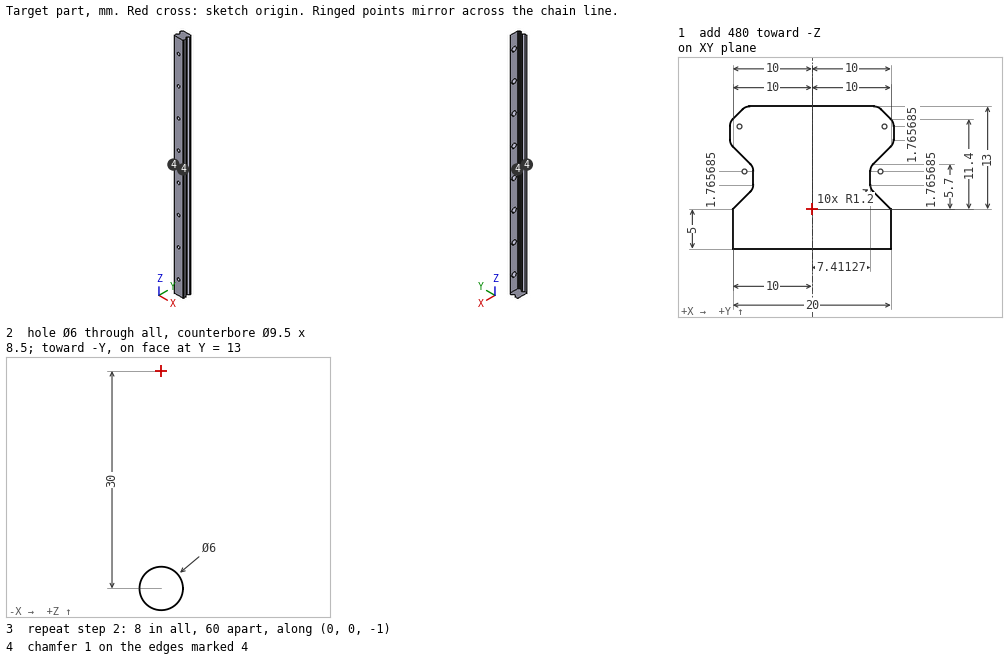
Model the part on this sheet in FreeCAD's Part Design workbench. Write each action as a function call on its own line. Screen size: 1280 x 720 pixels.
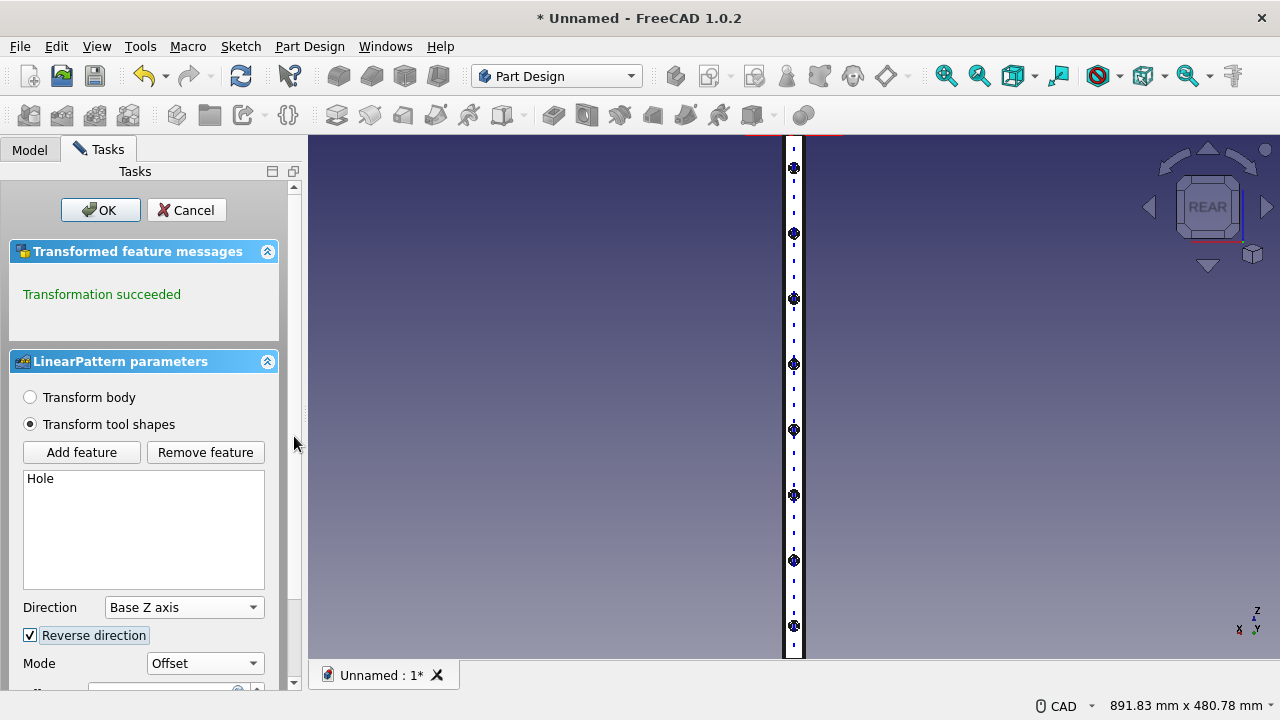
click(101, 210)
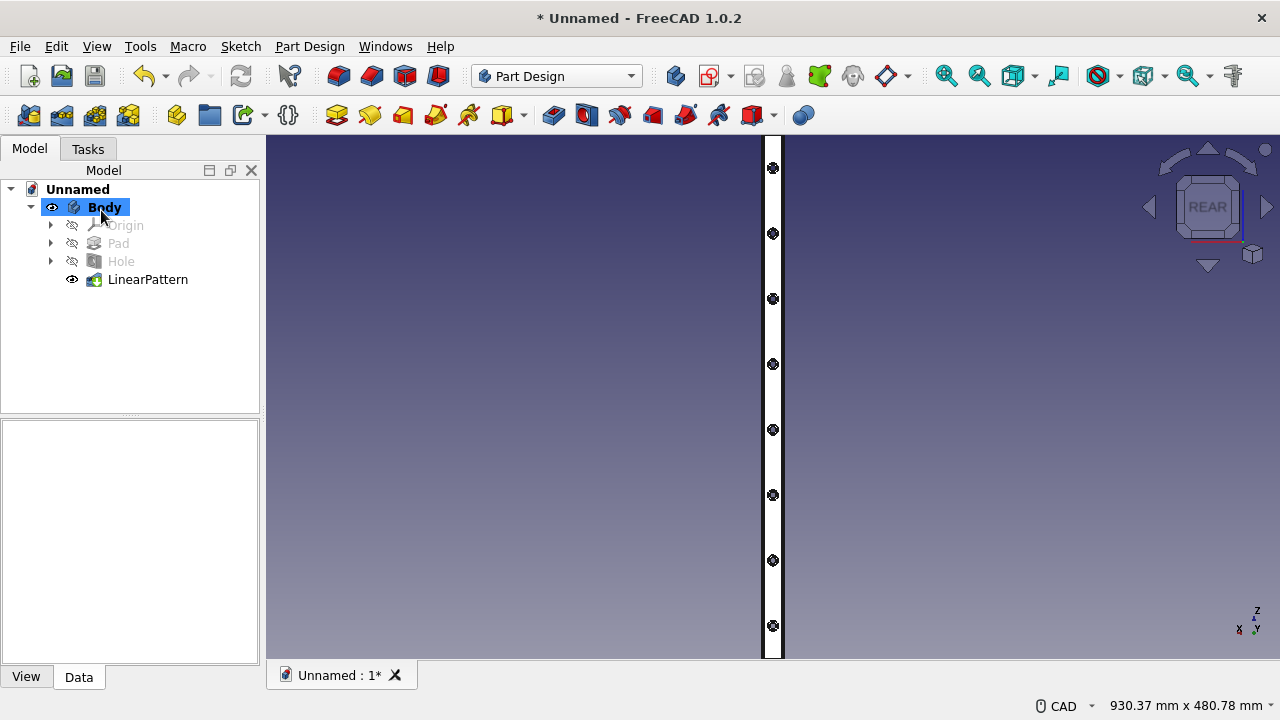
click(947, 76)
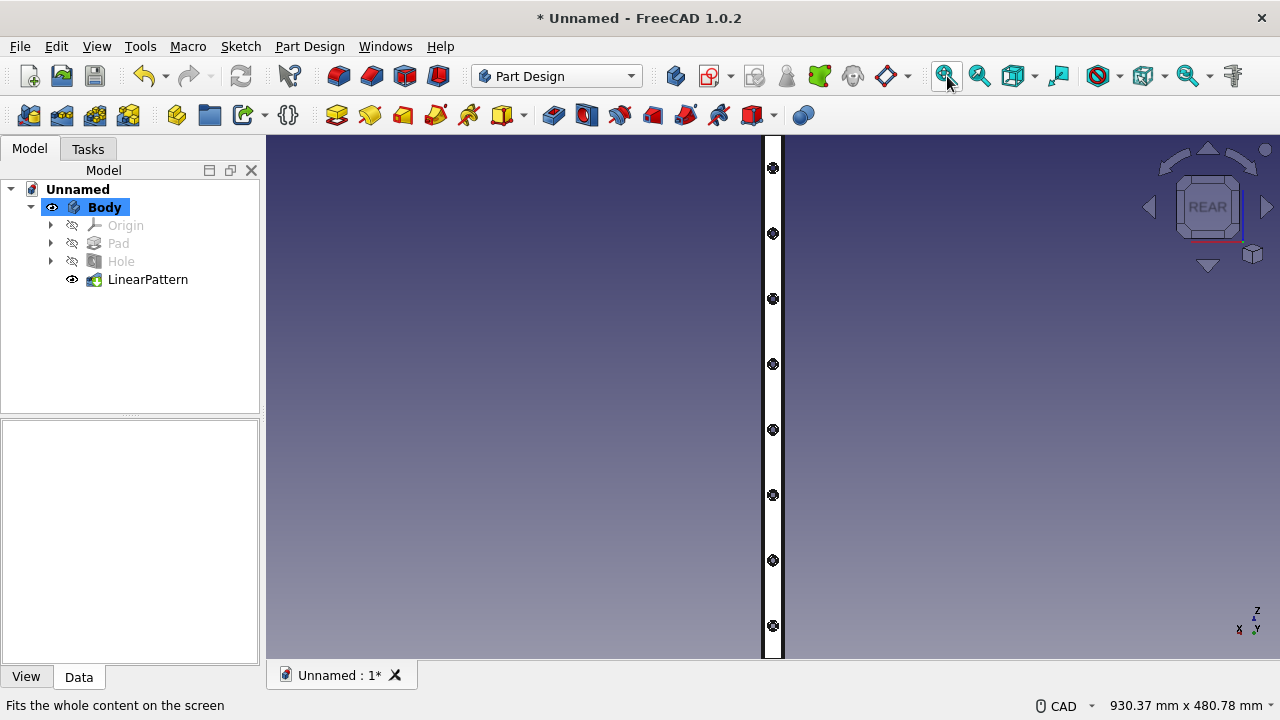
key(0)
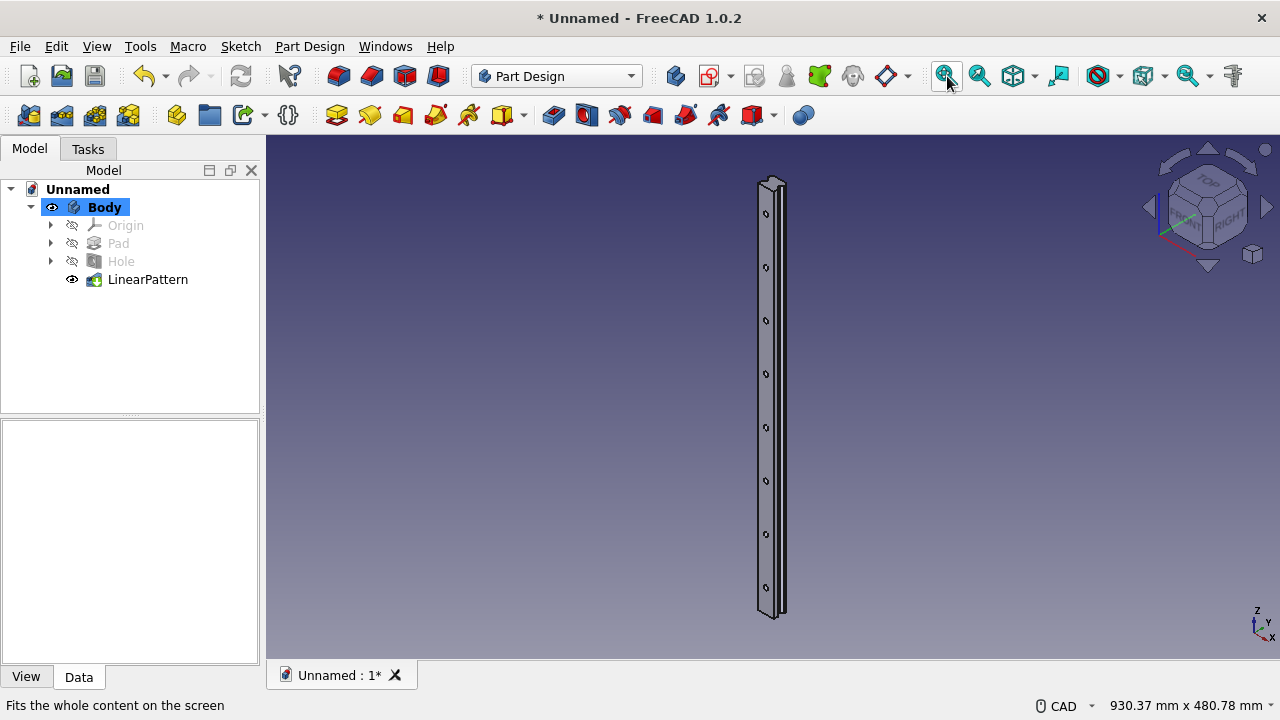
click(774, 404)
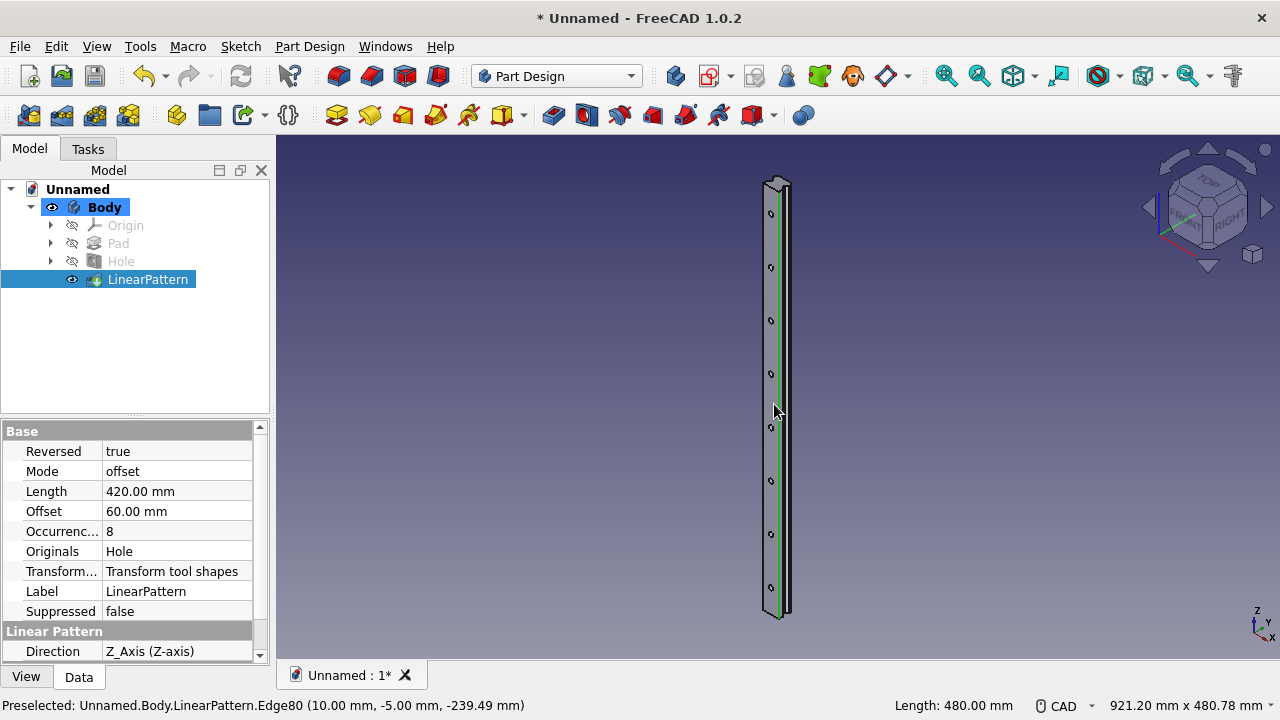
key(2)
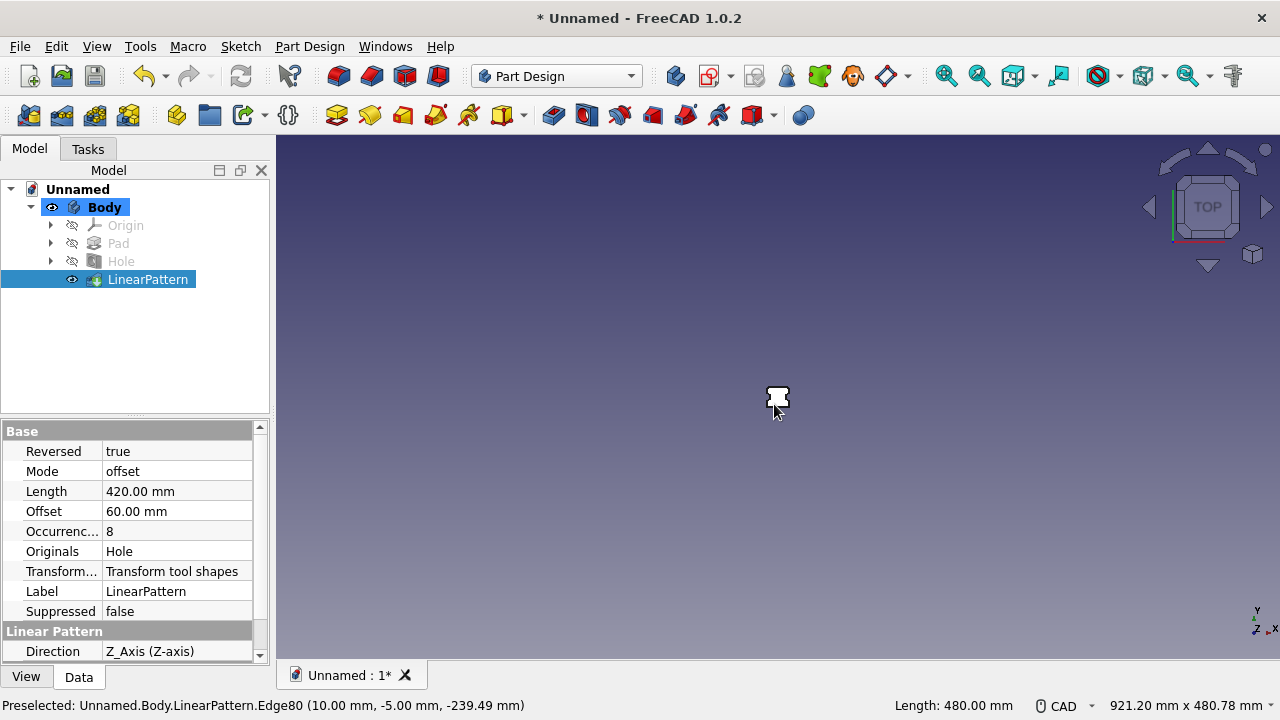
key(v)
key(f)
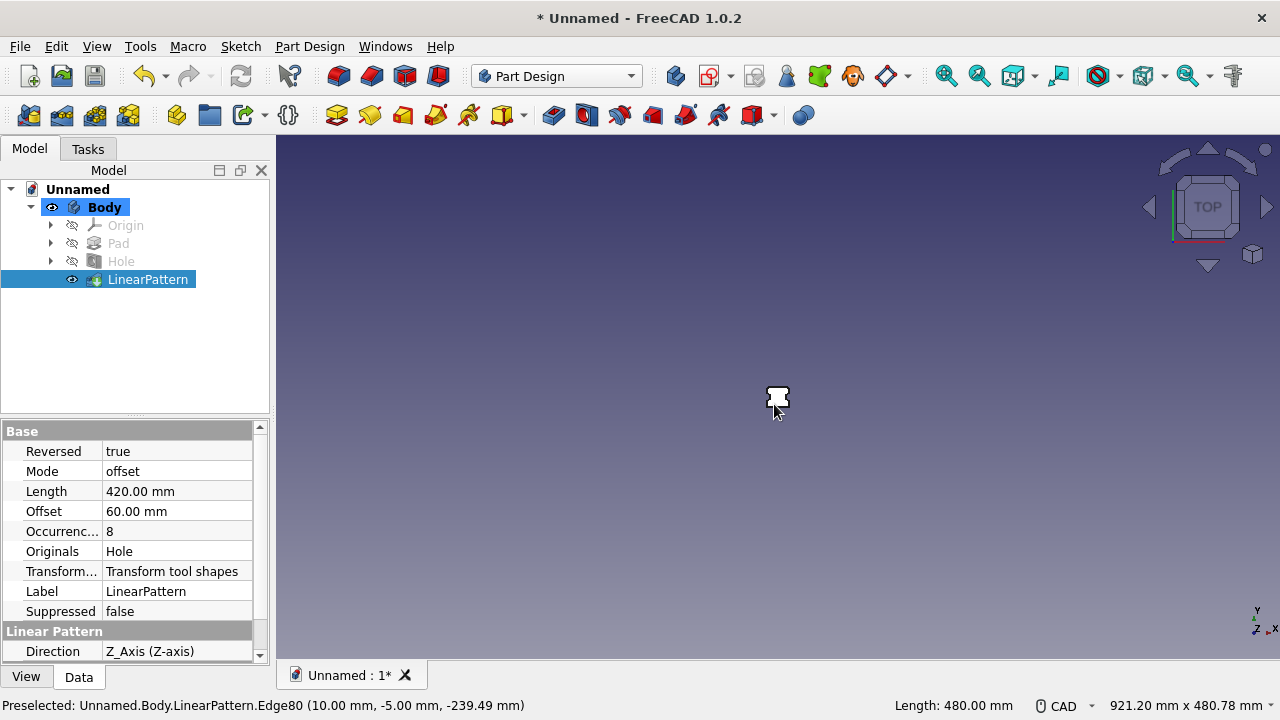
key(1)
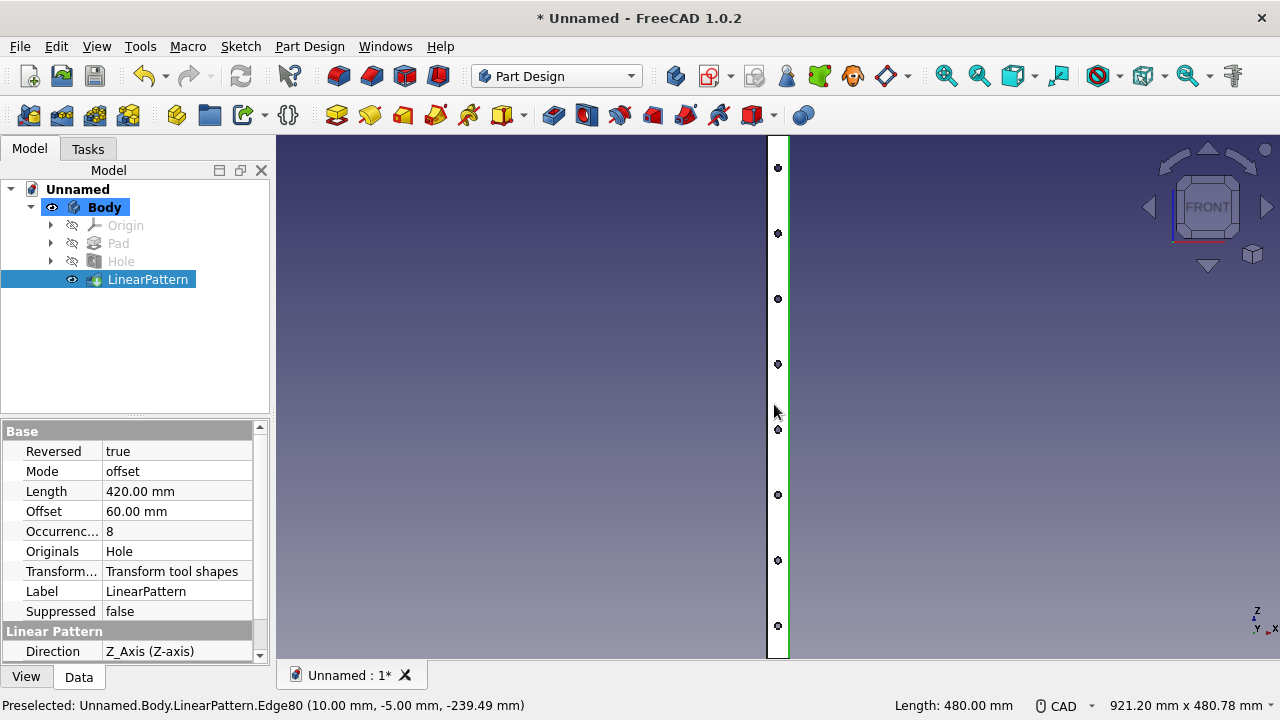
key(v)
key(f)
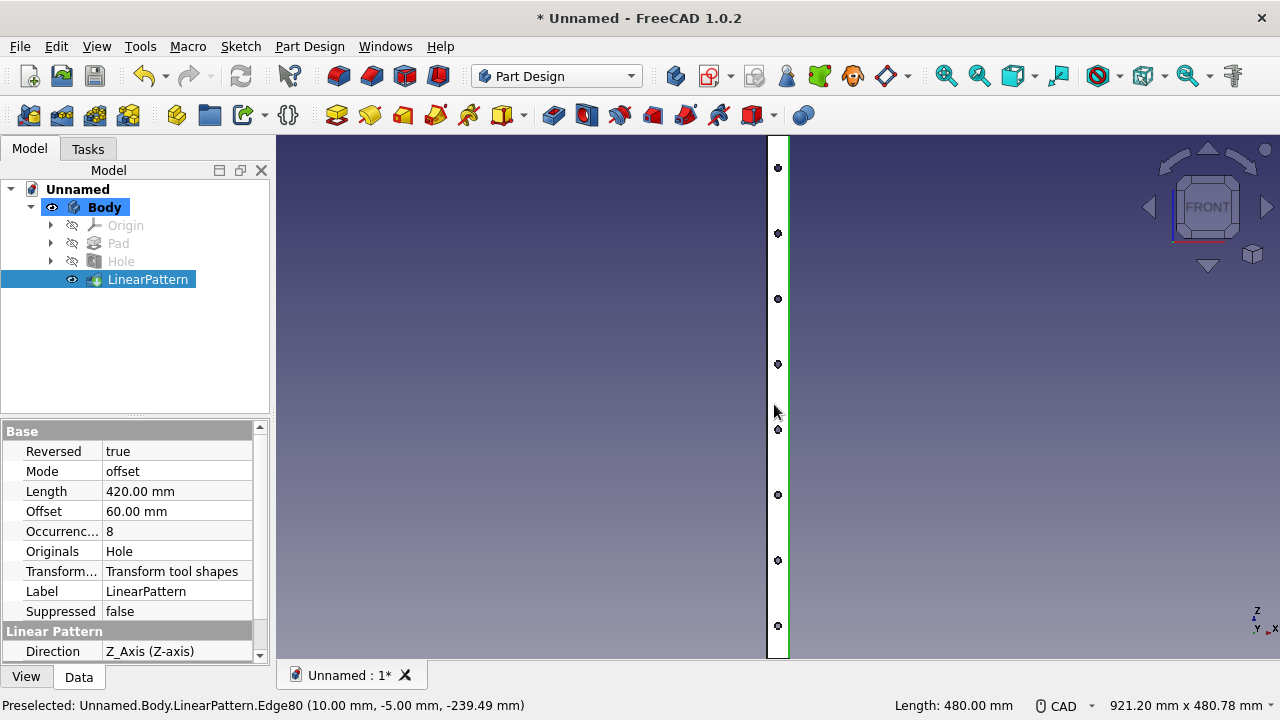
click(767, 396, ctrl)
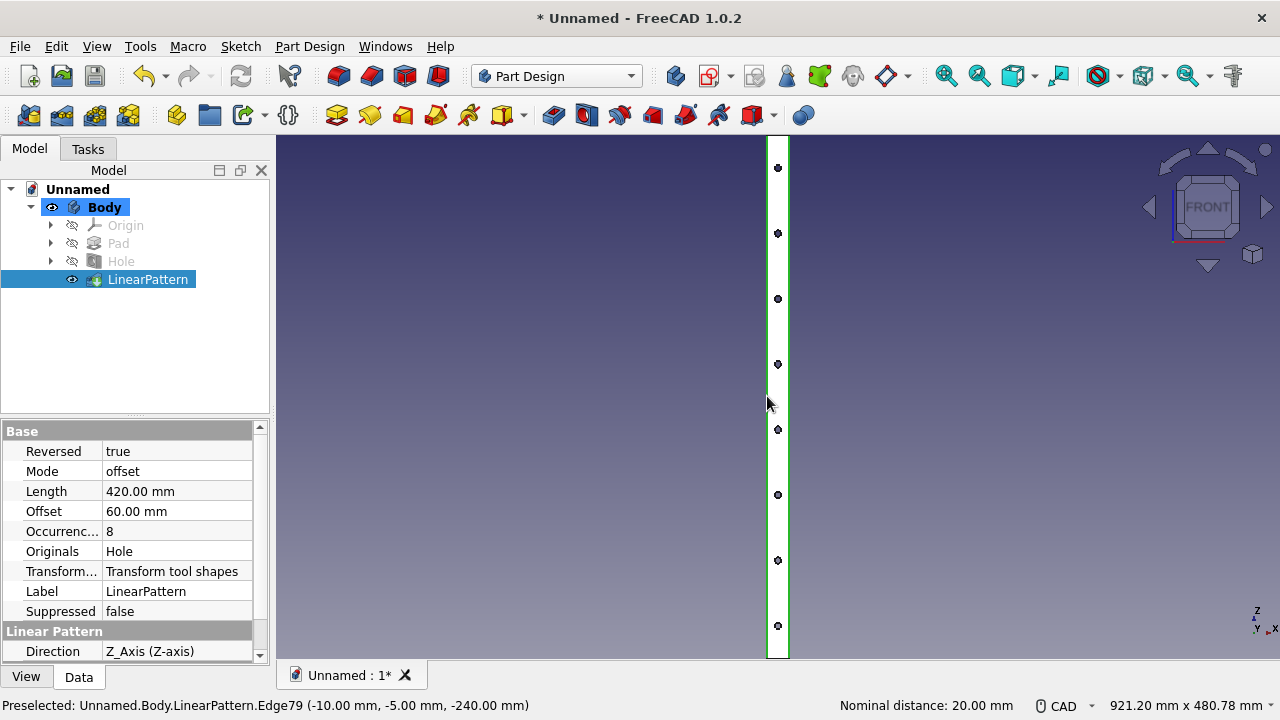
click(372, 76)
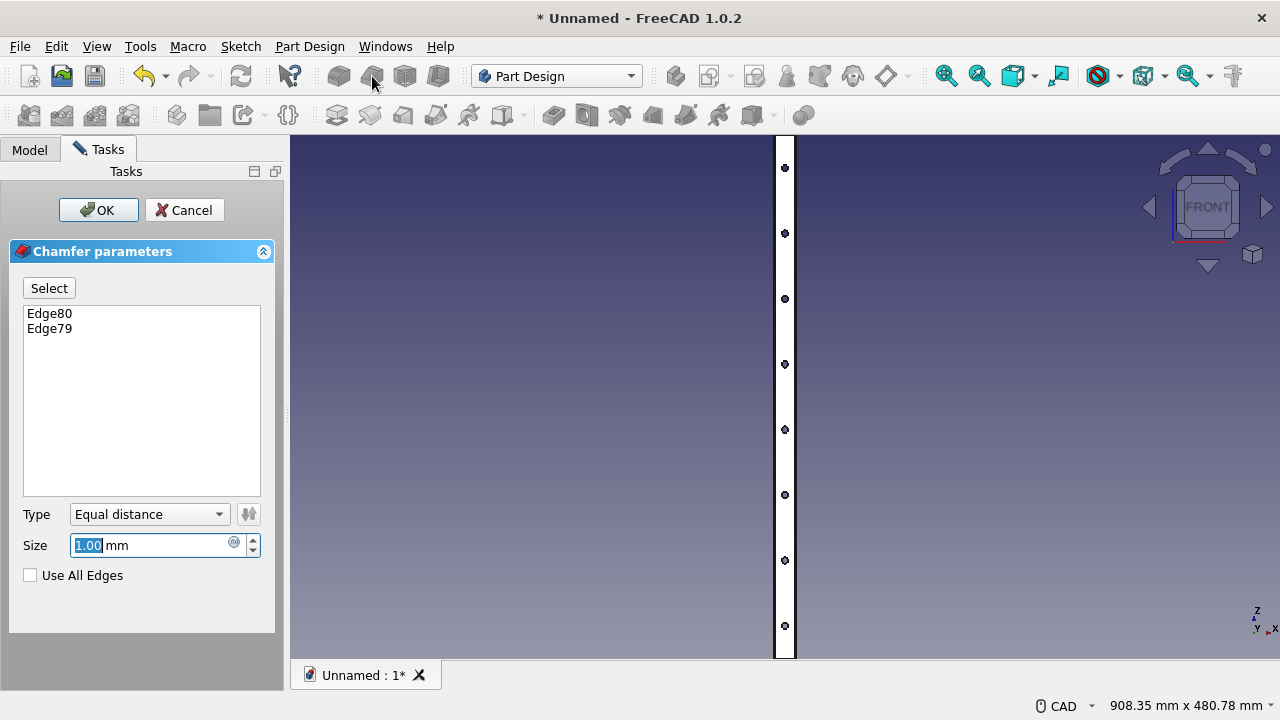
text(1)
key(Tab)